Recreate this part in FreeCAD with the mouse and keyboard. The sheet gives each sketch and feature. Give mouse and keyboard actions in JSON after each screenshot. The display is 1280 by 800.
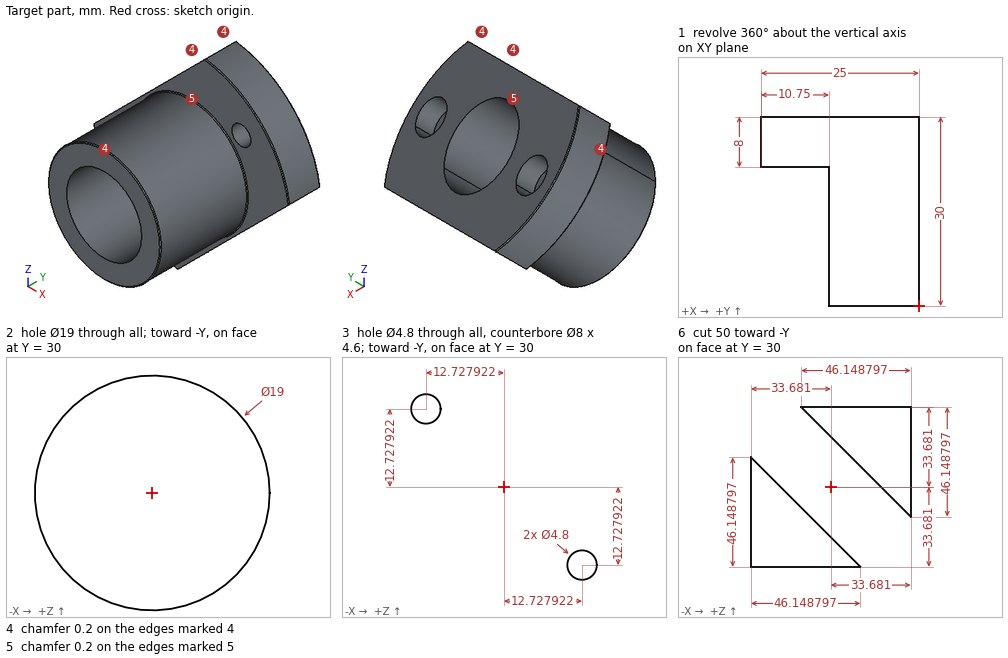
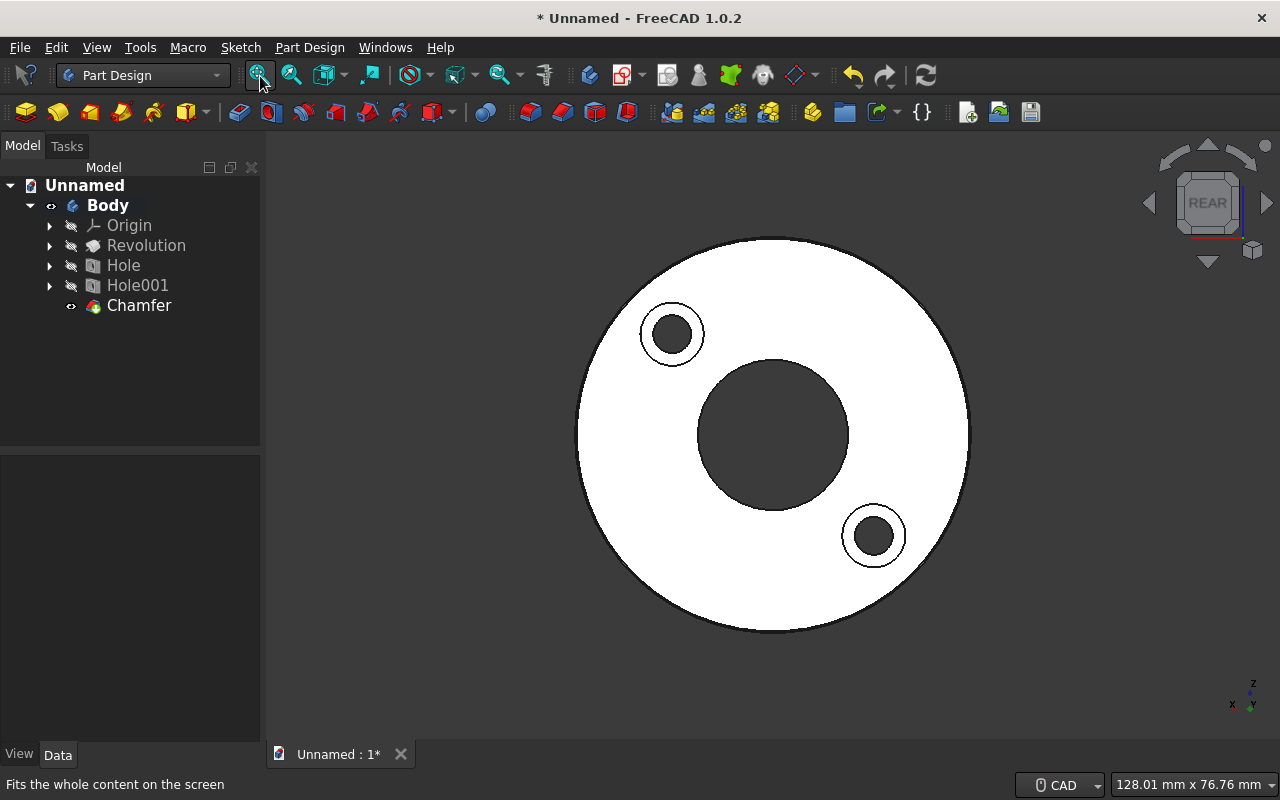
{"action": "key", "text": "6"}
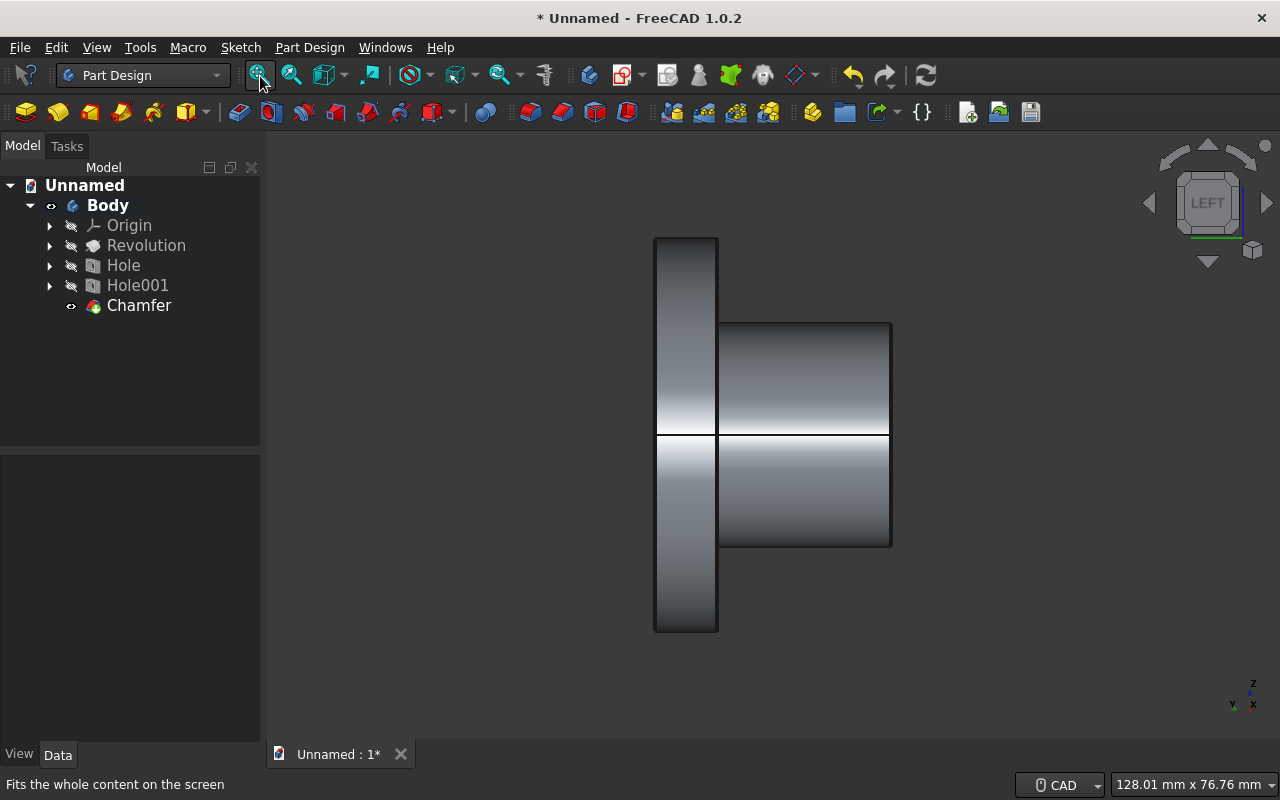
{"action": "key", "text": "v 3"}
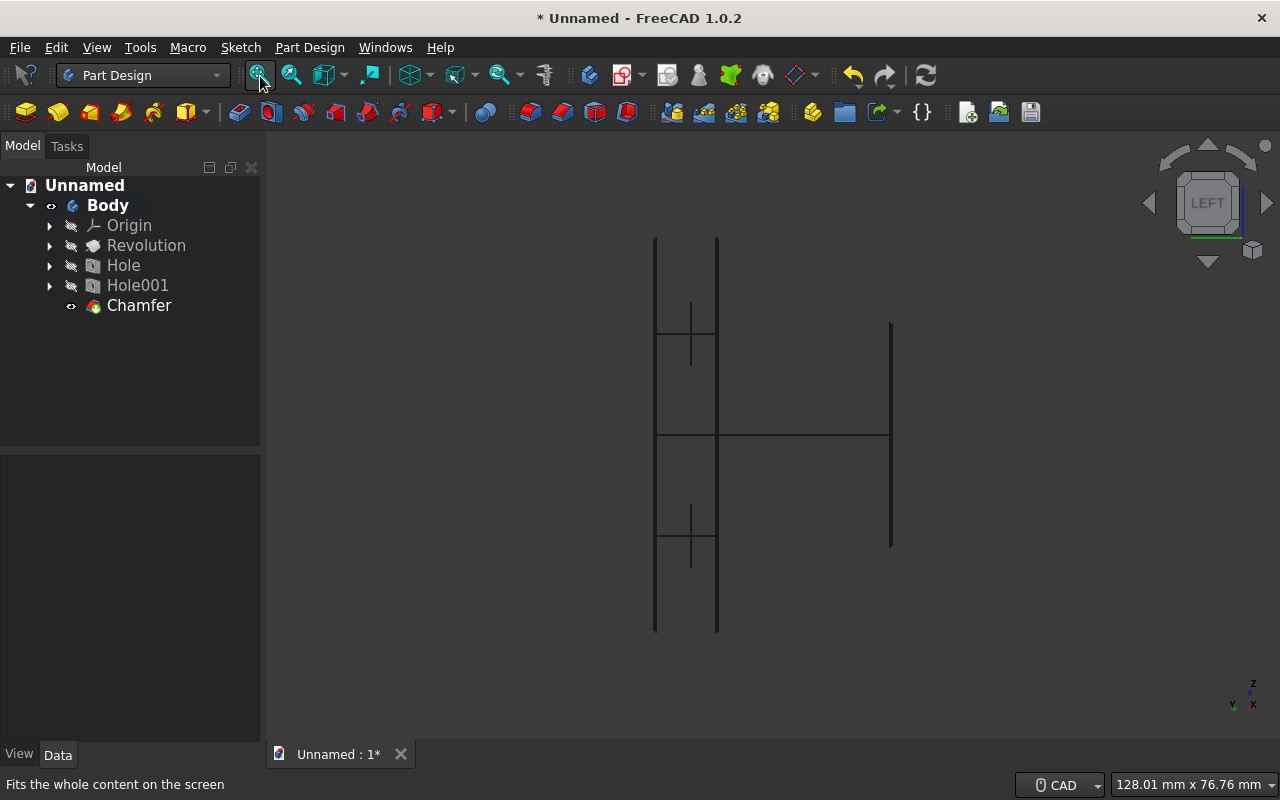
{"action": "key", "text": "0"}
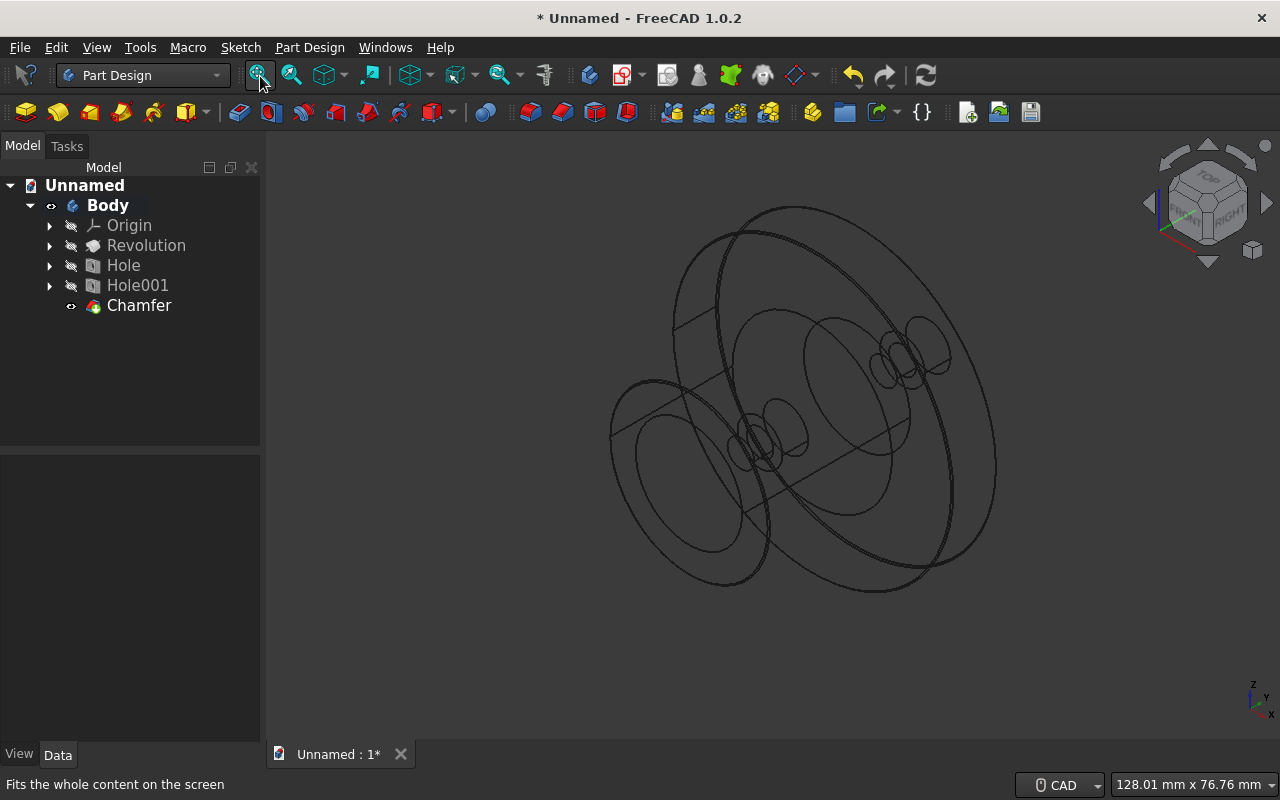
{"action": "left_click", "coordinate": [892, 457]}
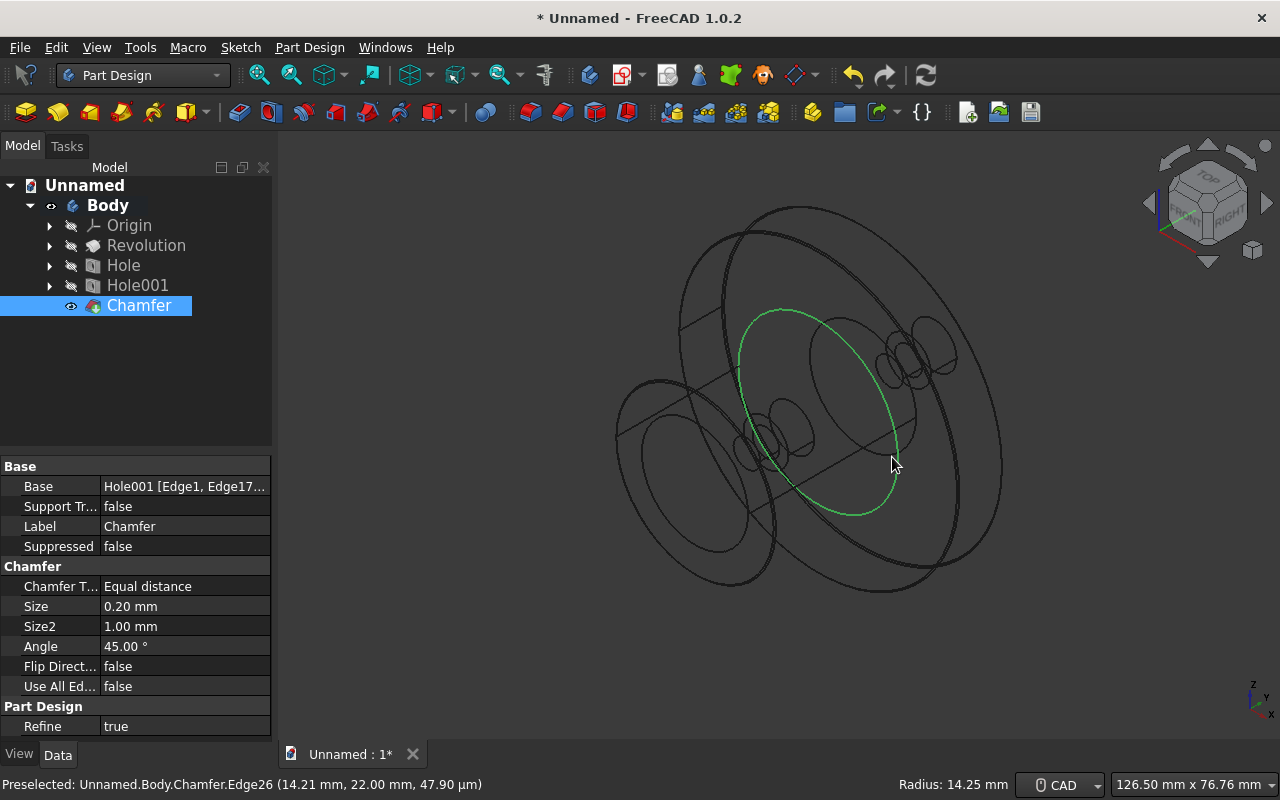
{"action": "key", "text": "v 1"}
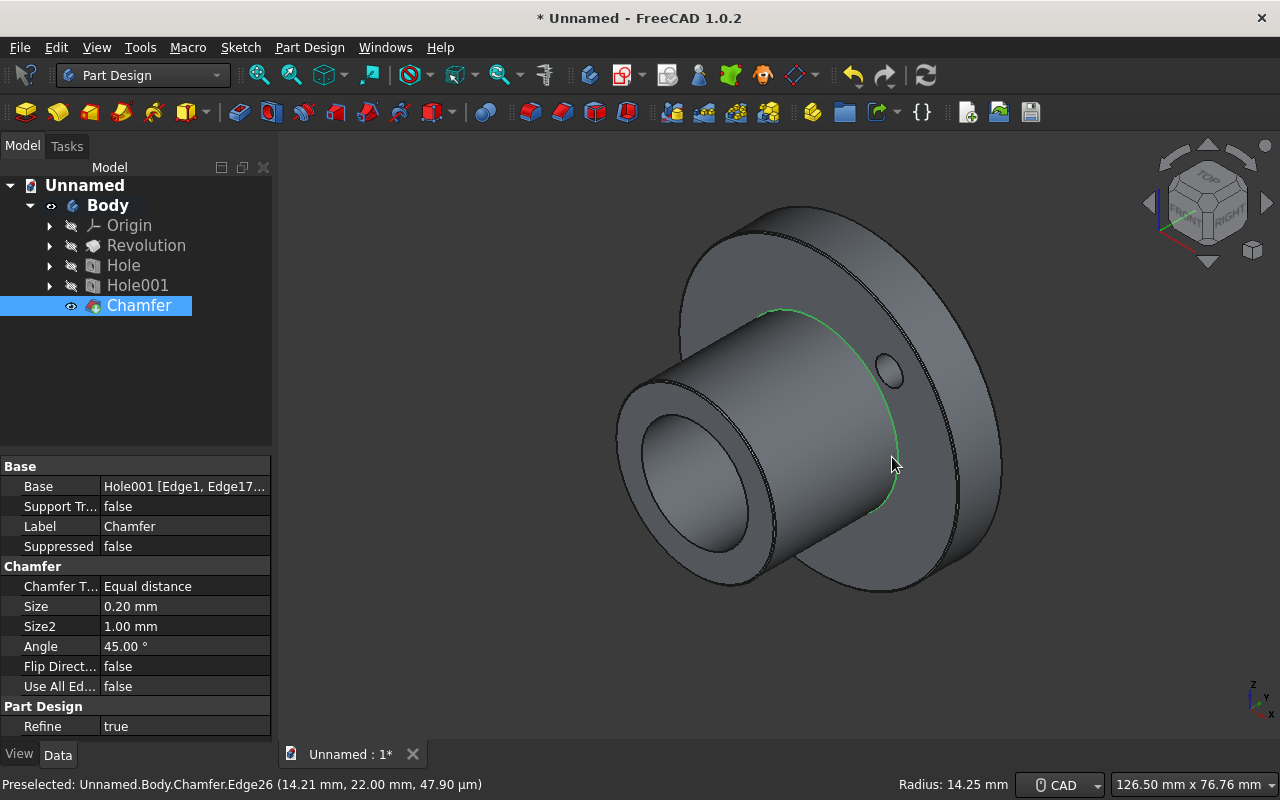
{"action": "left_click", "coordinate": [564, 112]}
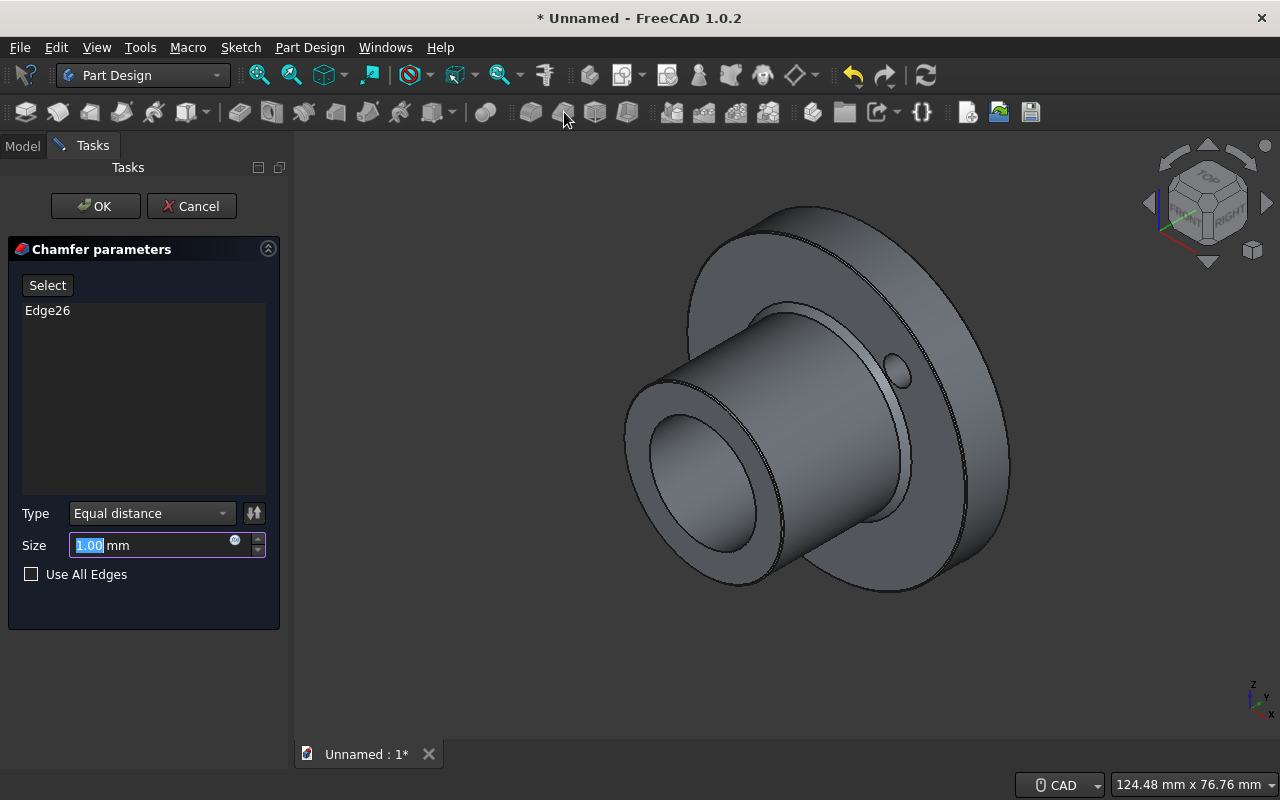
{"action": "type", "text": "0.2"}
{"action": "key", "text": "Tab"}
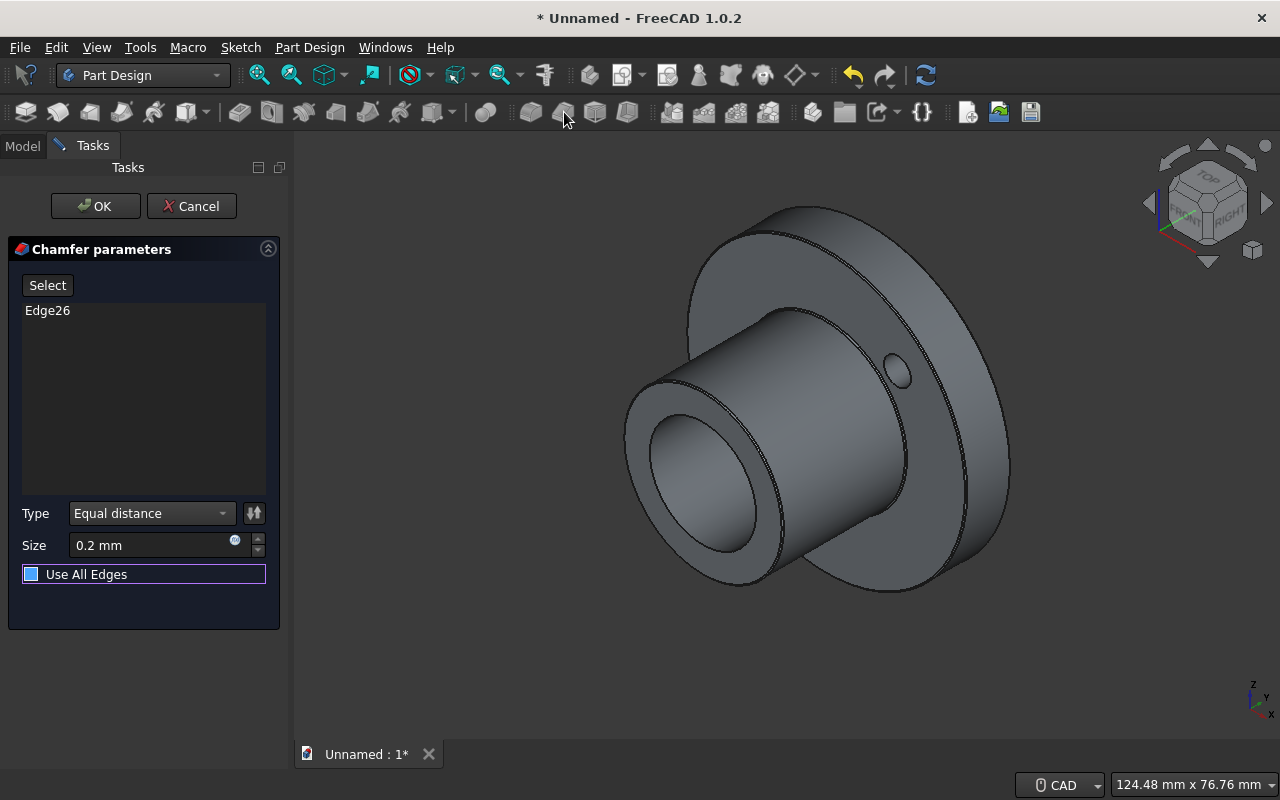
{"action": "left_click", "coordinate": [96, 206]}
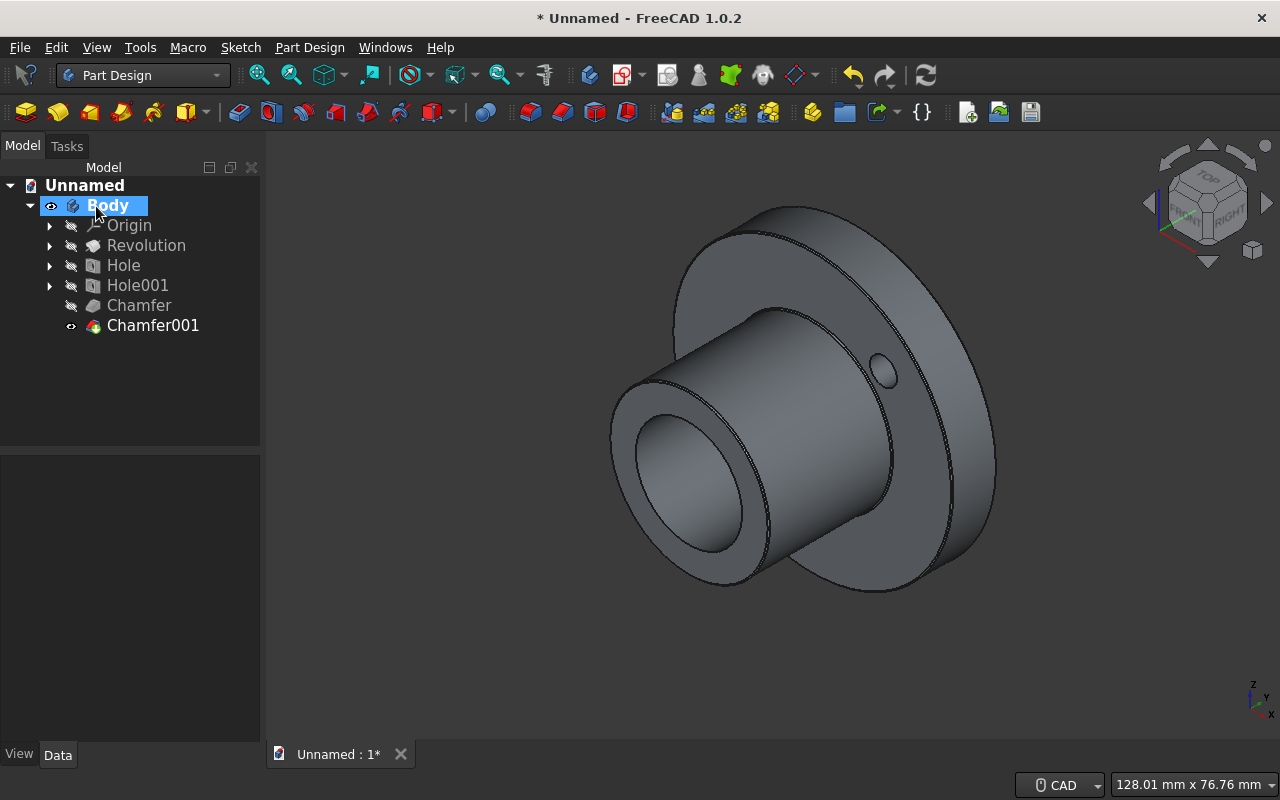
{"action": "key", "text": "4"}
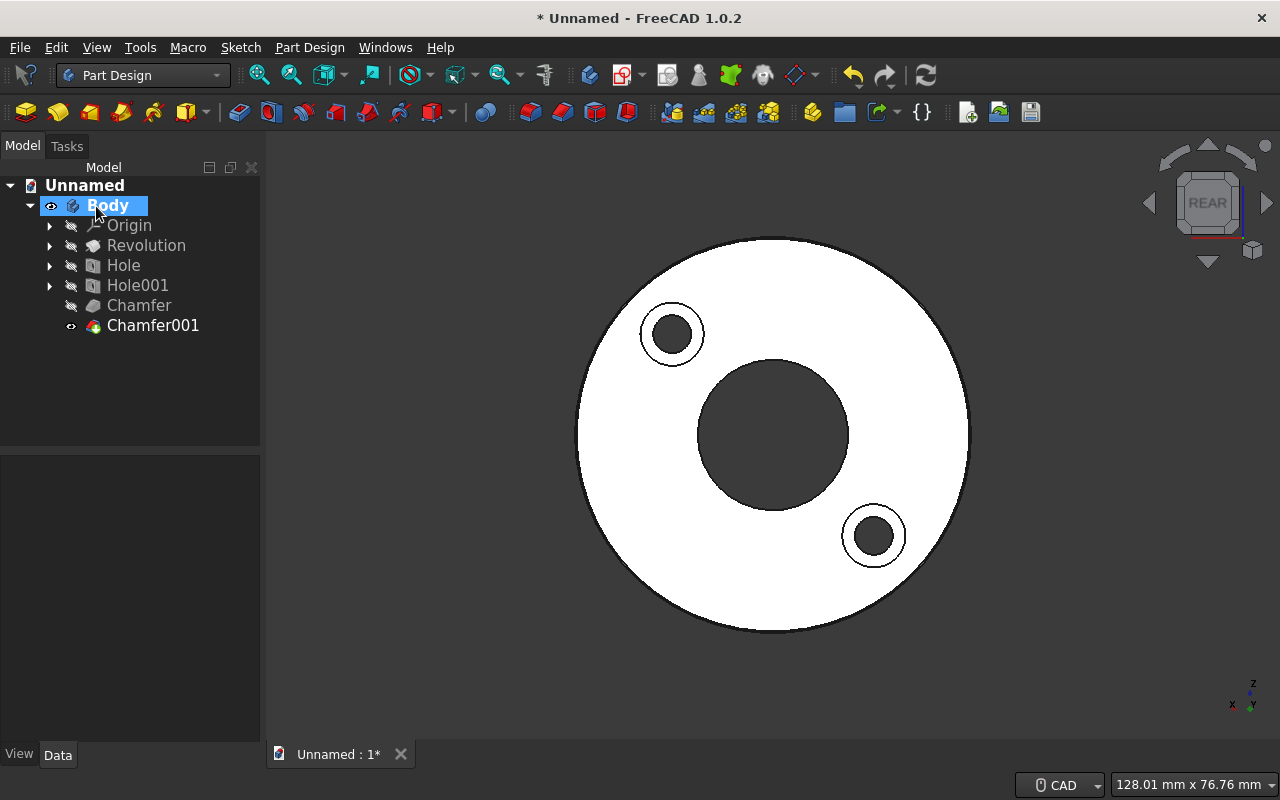
{"action": "left_click", "coordinate": [661, 490]}